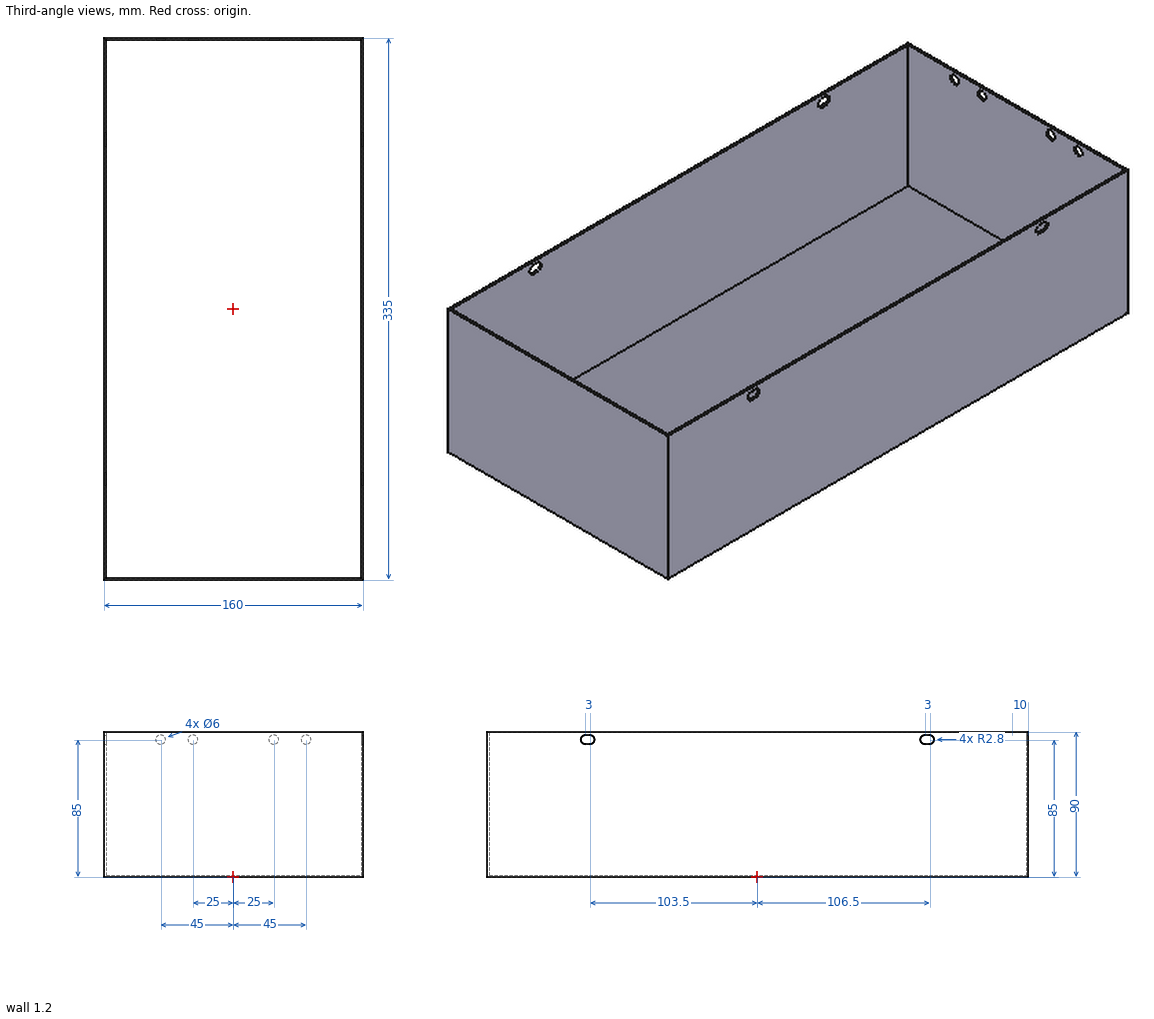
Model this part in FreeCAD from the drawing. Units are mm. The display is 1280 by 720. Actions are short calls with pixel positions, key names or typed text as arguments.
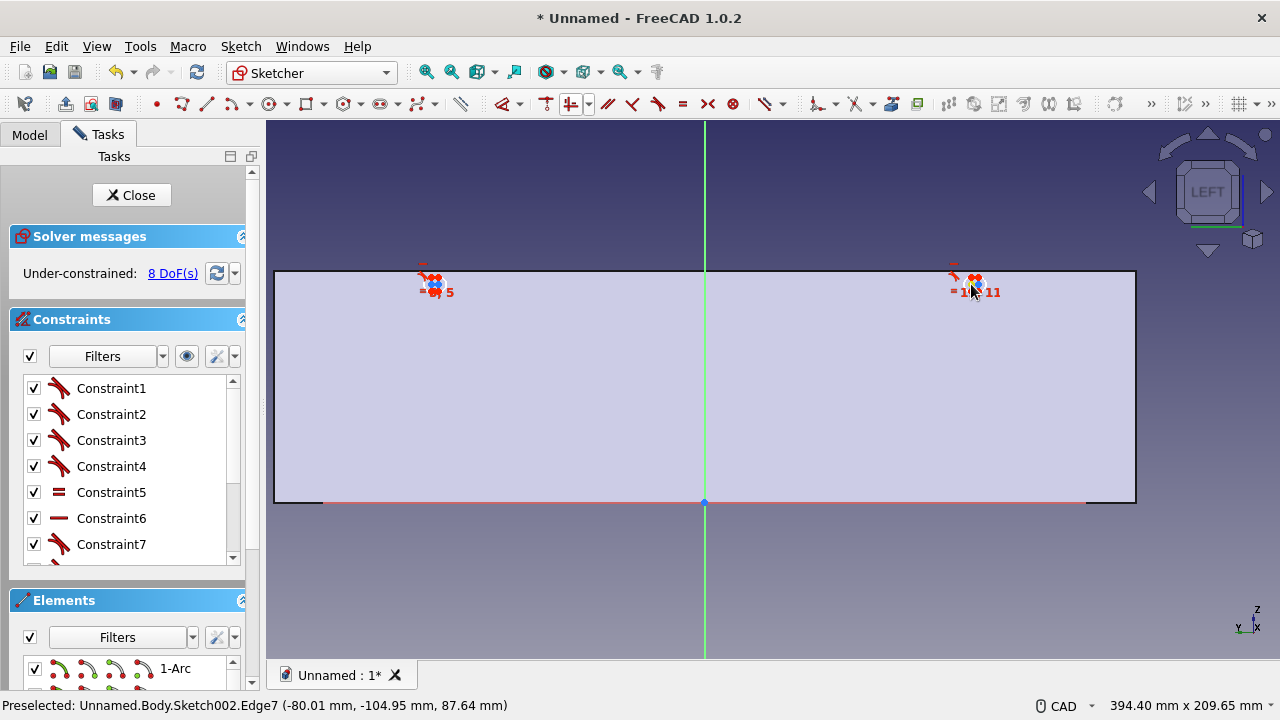
scroll(425, 280, up, 4)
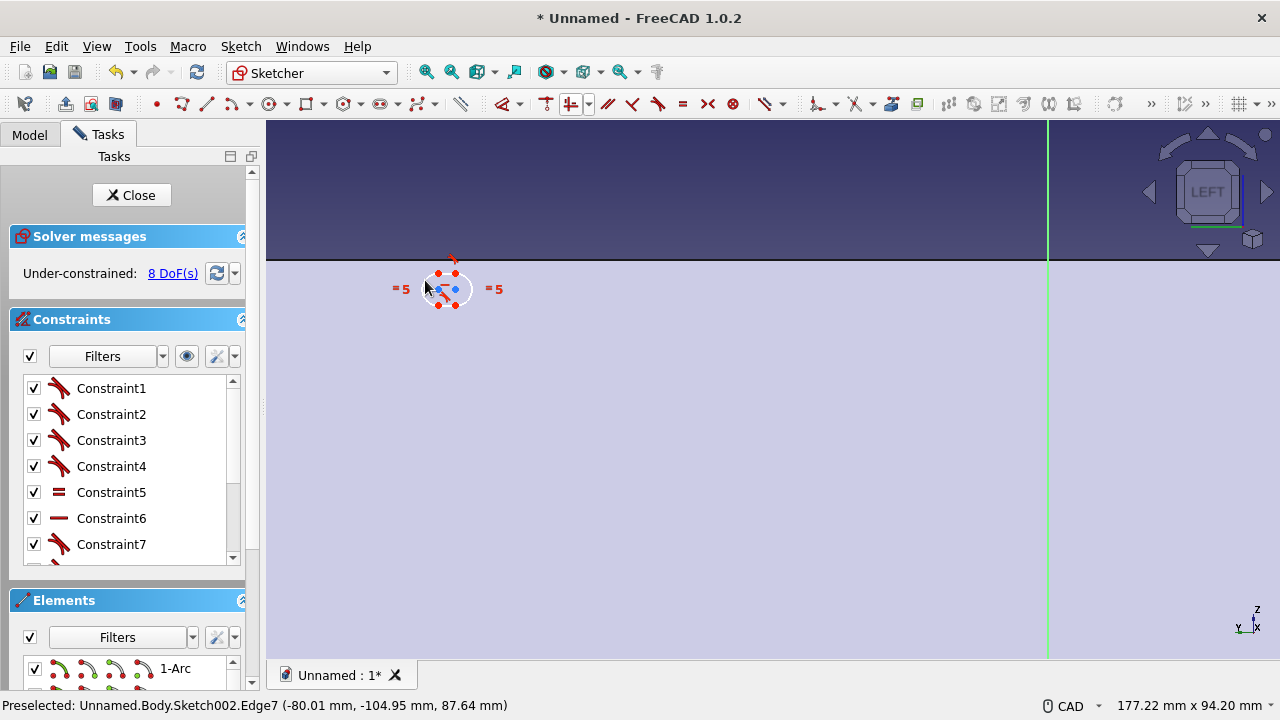
click(425, 280)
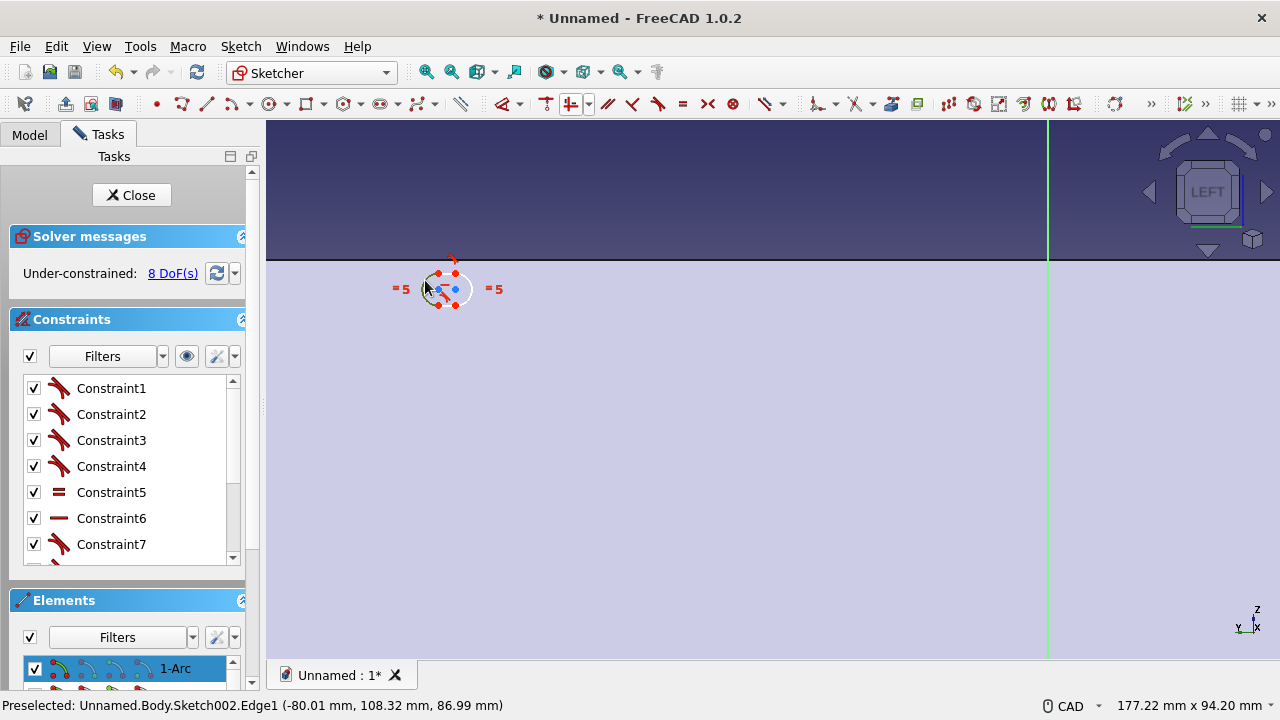
scroll(424, 280, down, 4)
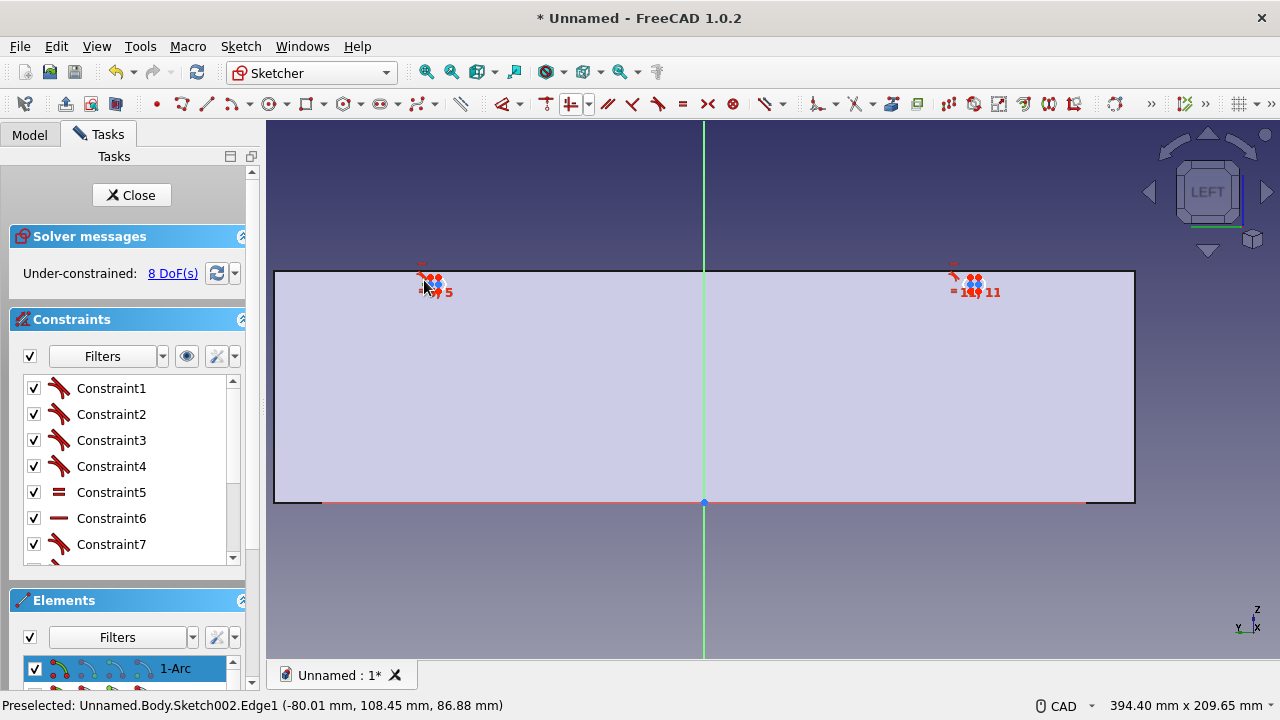
scroll(965, 280, up, 4)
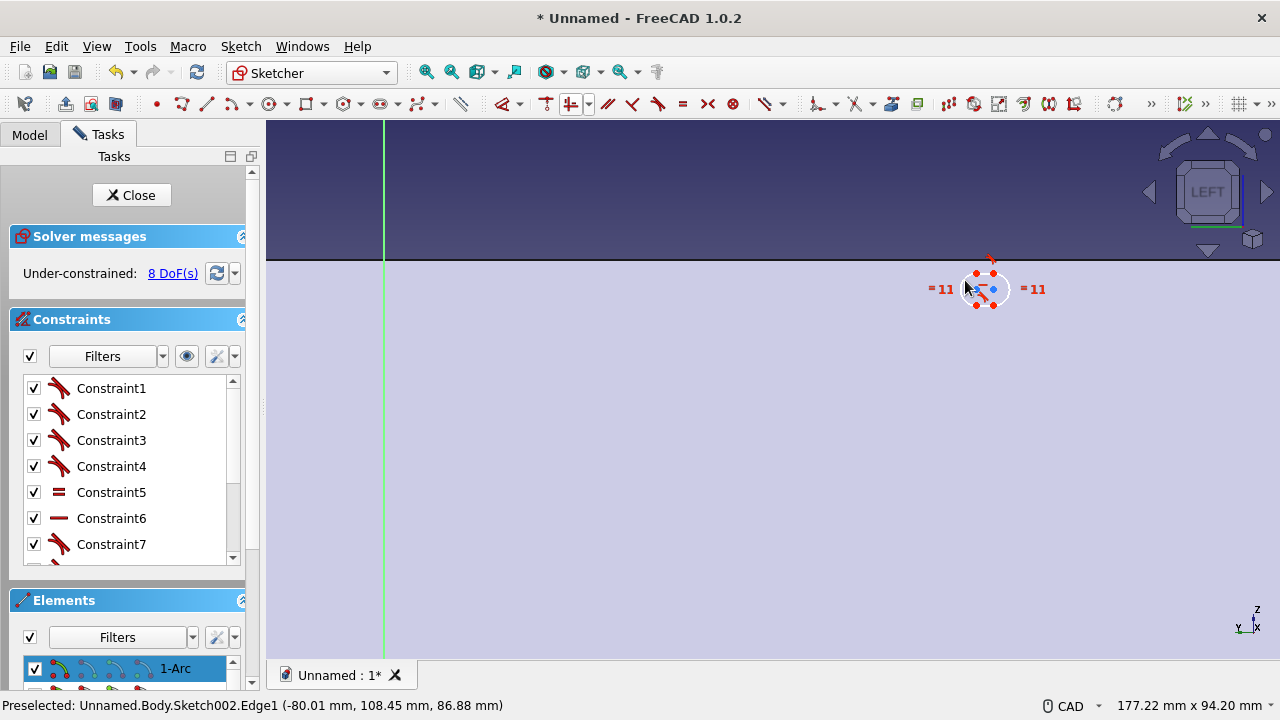
click(964, 280)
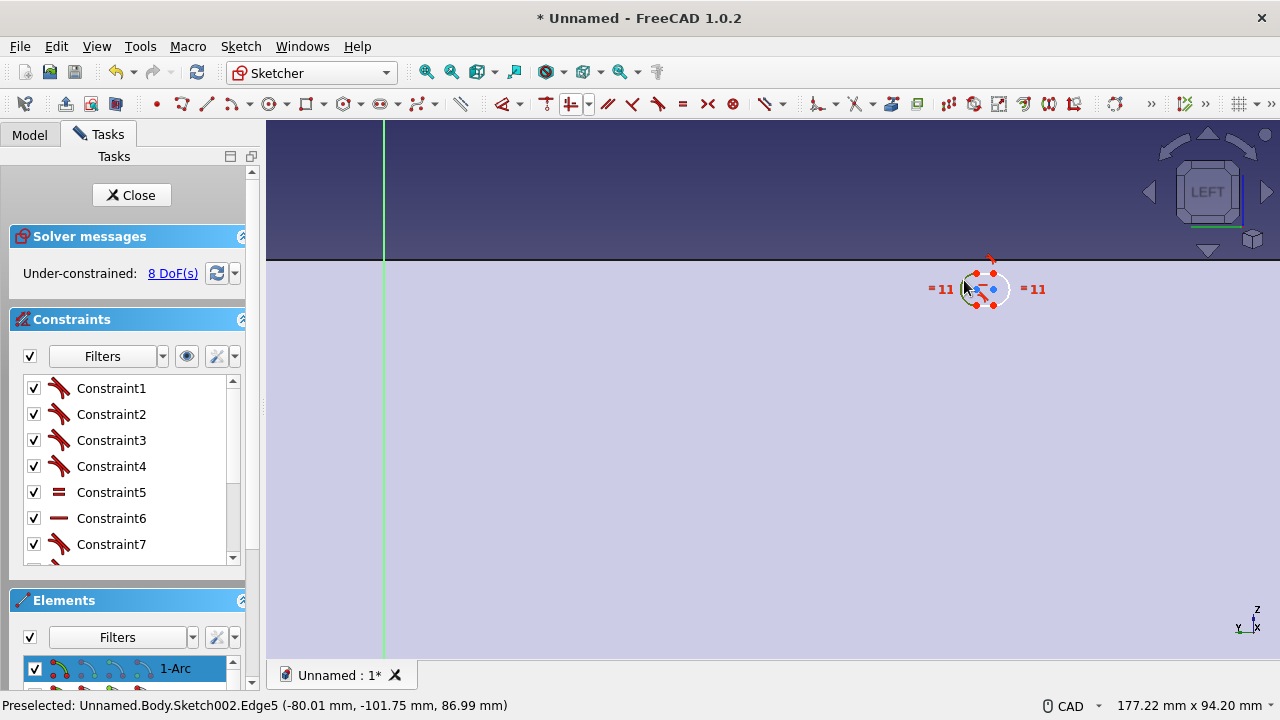
click(683, 104)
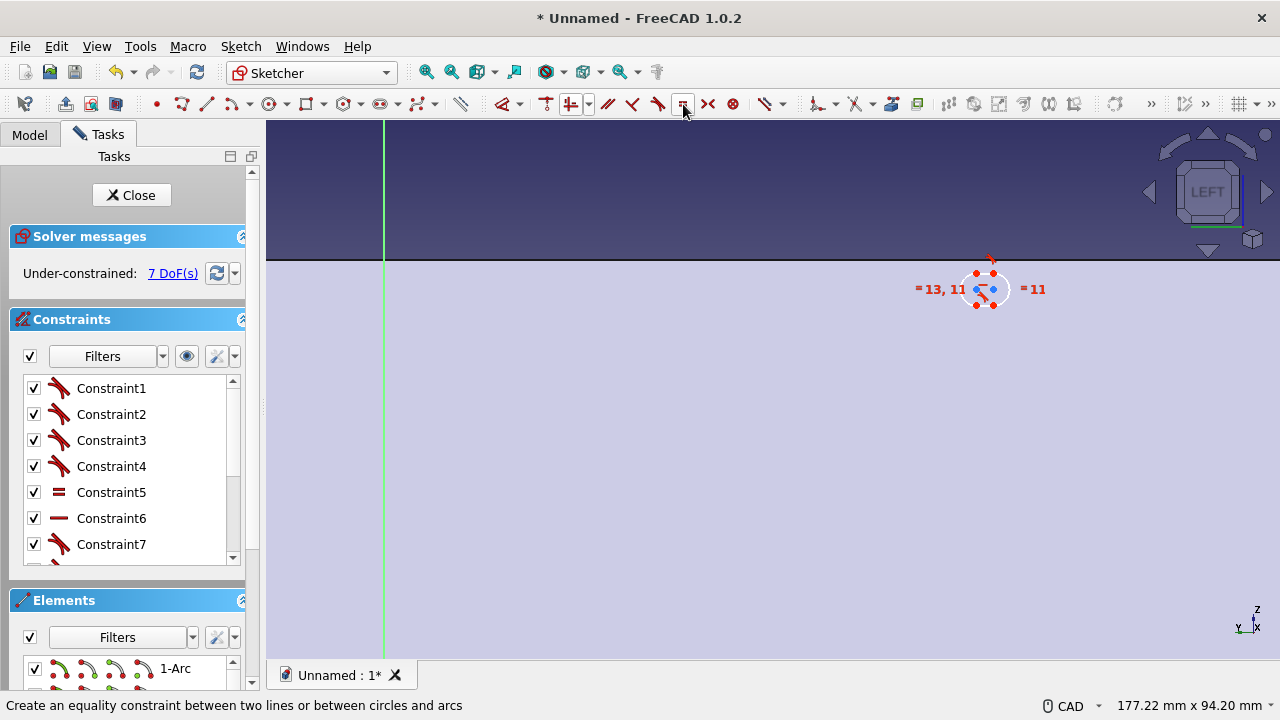
key(d)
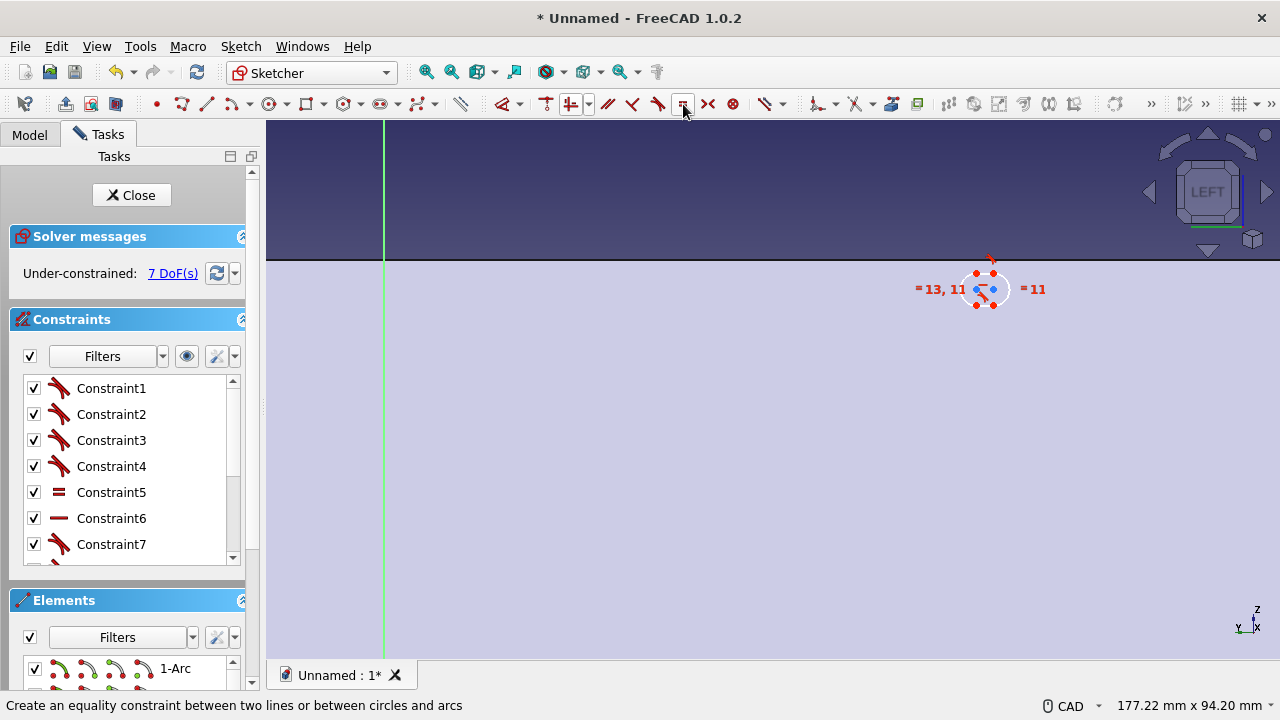
scroll(966, 280, down, 4)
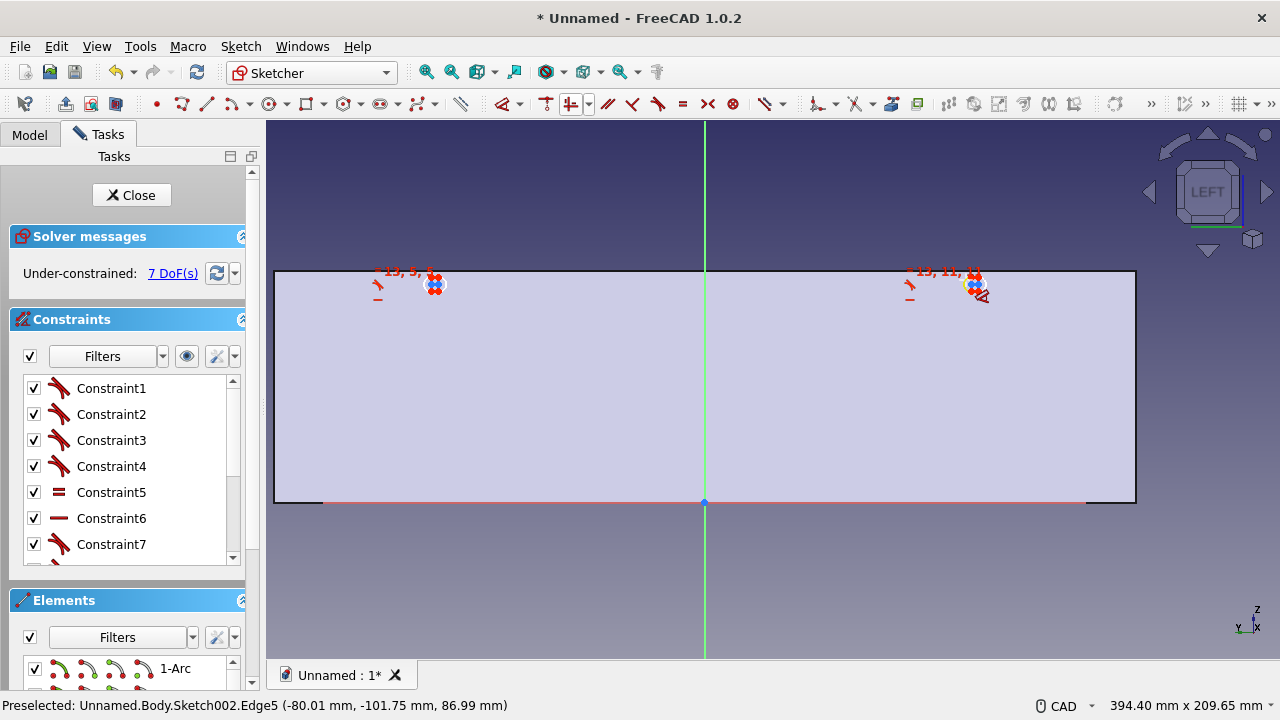
scroll(425, 280, up, 9)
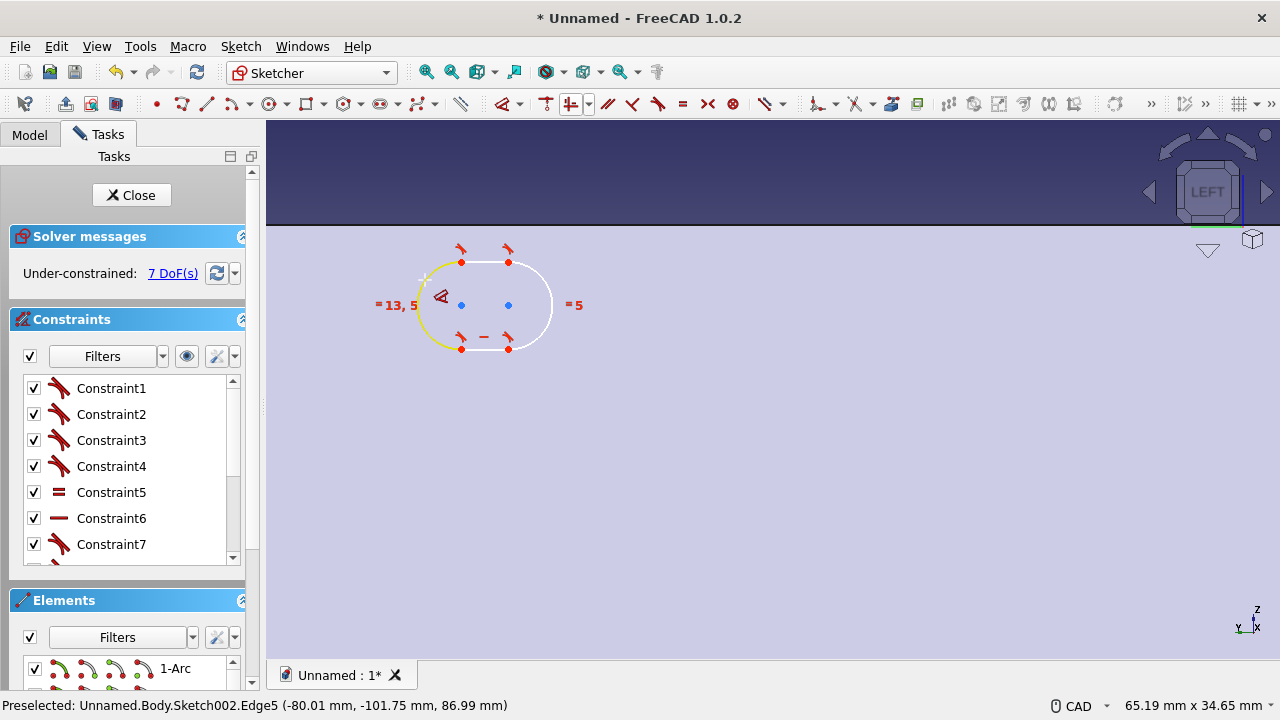
click(426, 280)
click(400, 261)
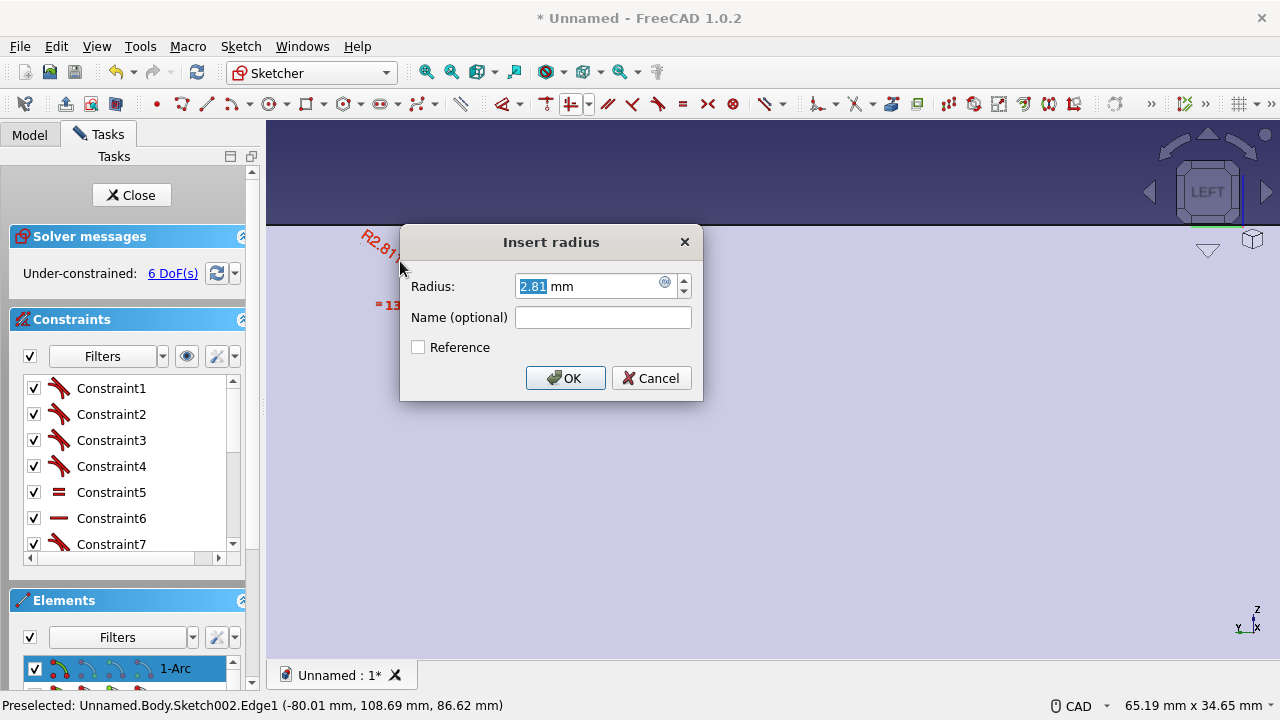
text(2.8)
key(Return)